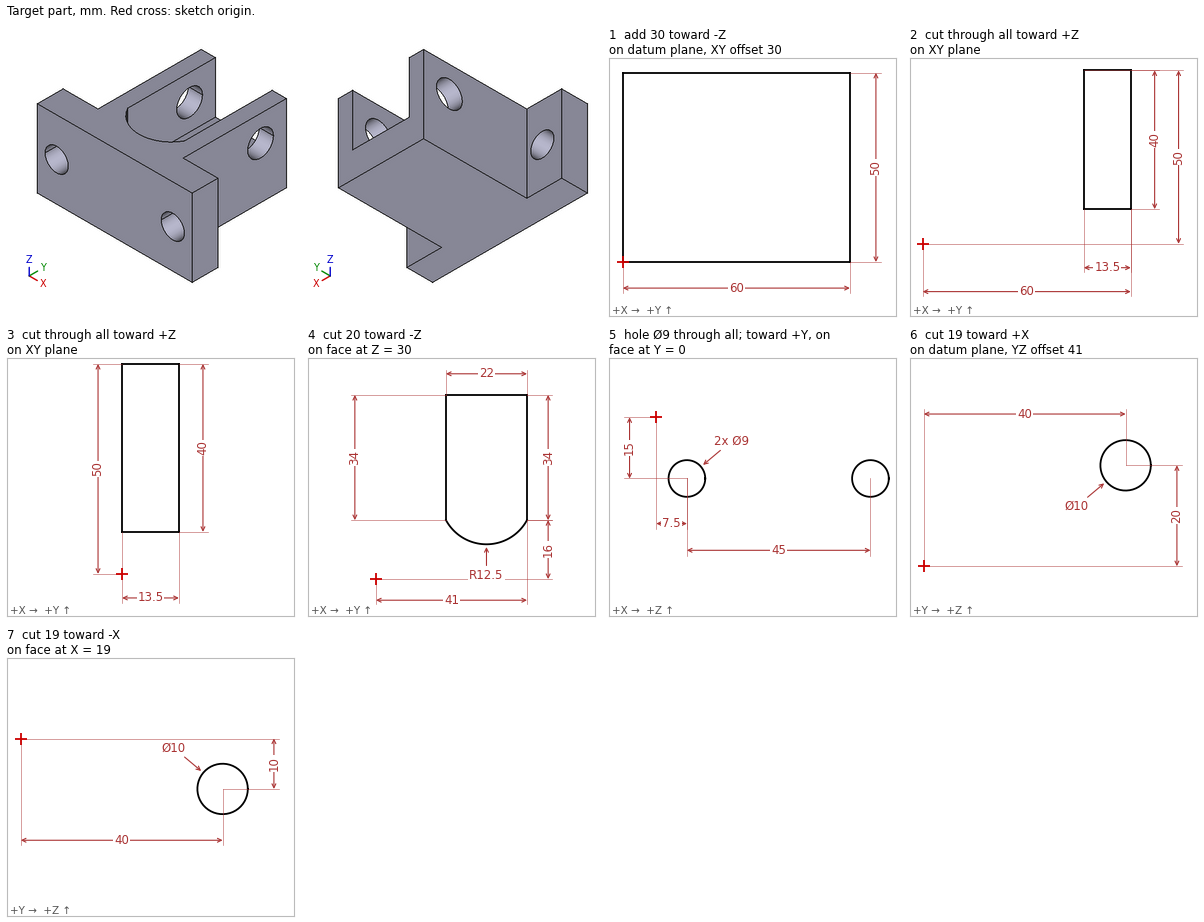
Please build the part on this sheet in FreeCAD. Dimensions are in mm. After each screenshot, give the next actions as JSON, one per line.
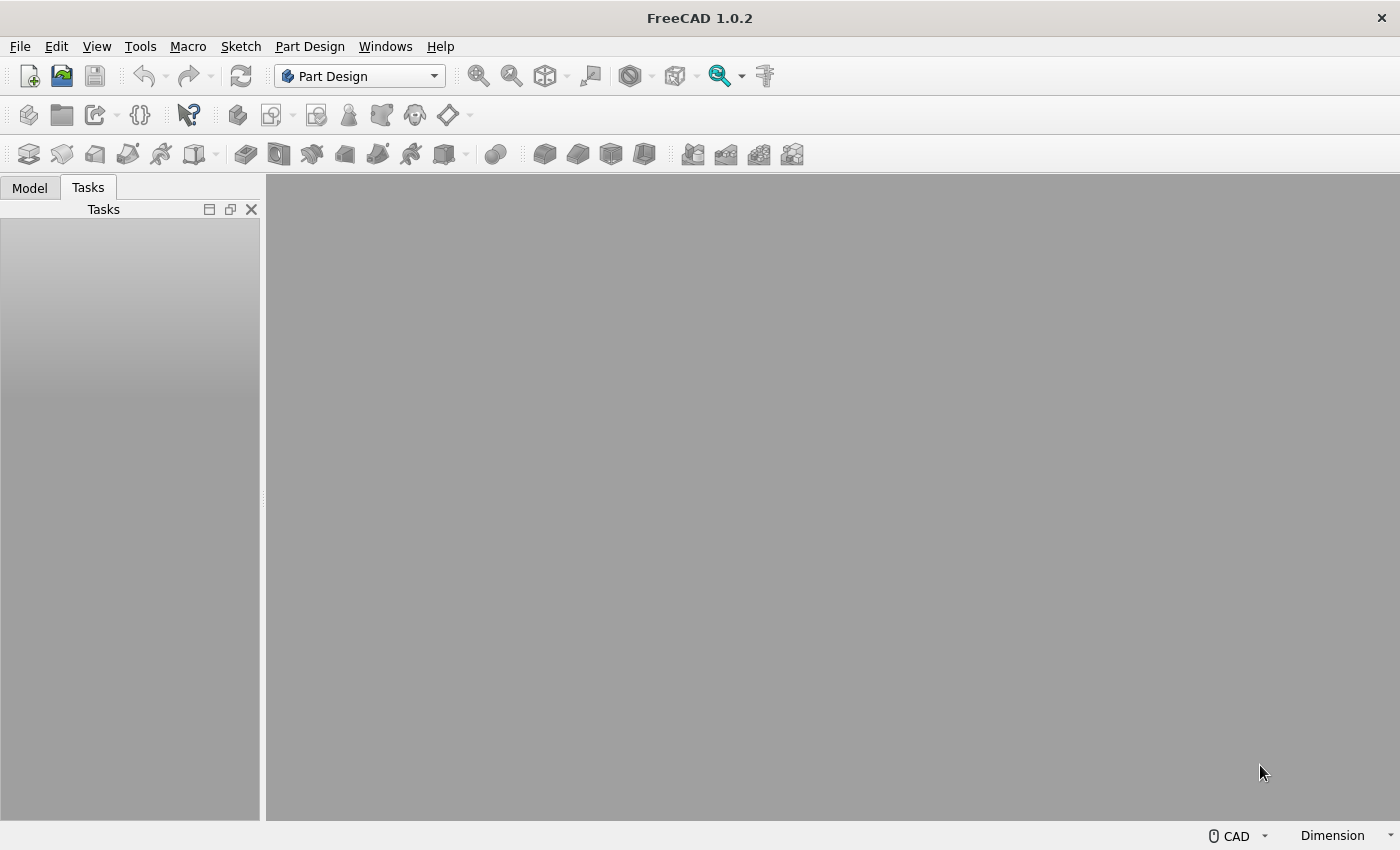
{"action": "key", "text": "ctrl+n"}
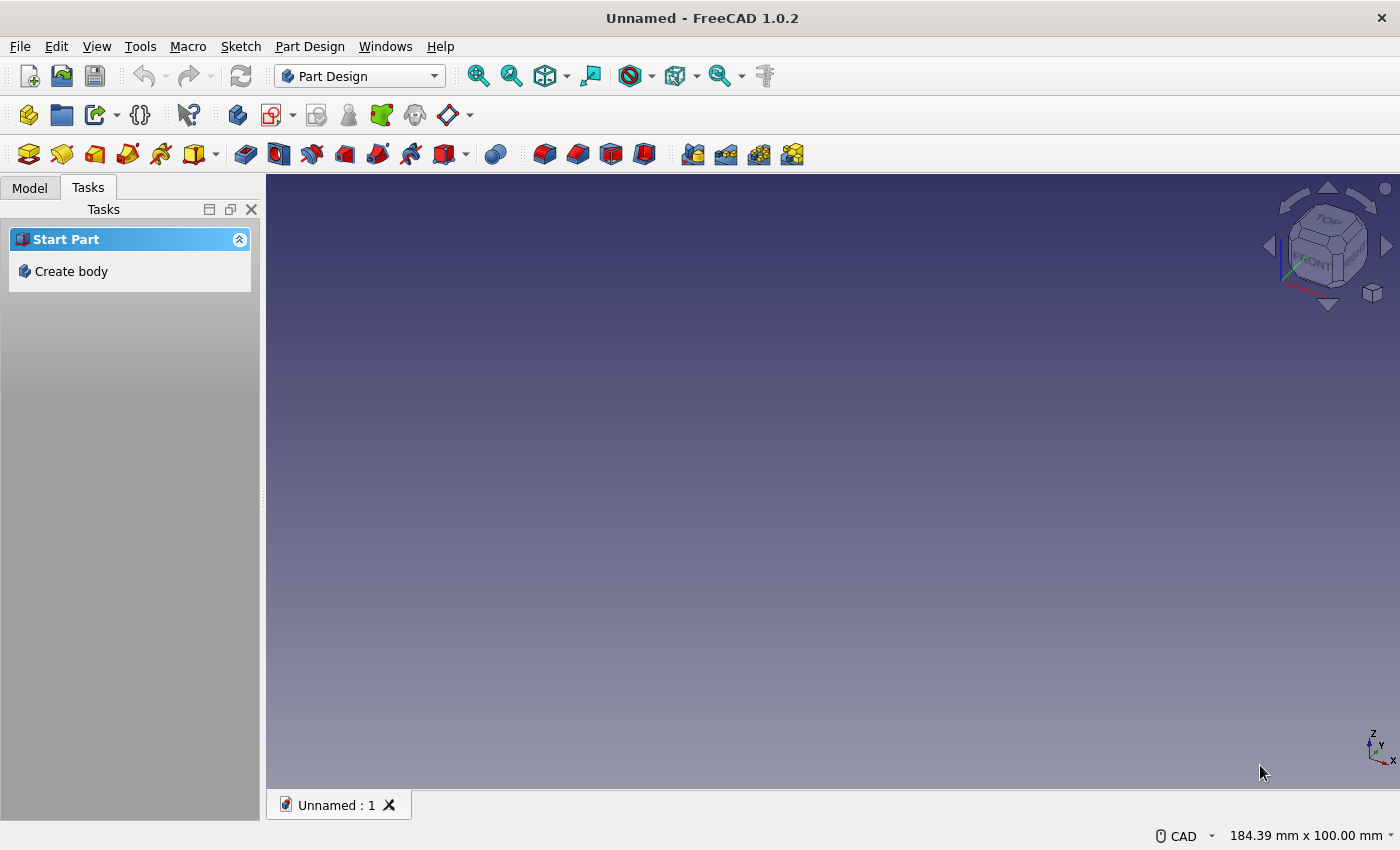
{"action": "left_click", "coordinate": [238, 116]}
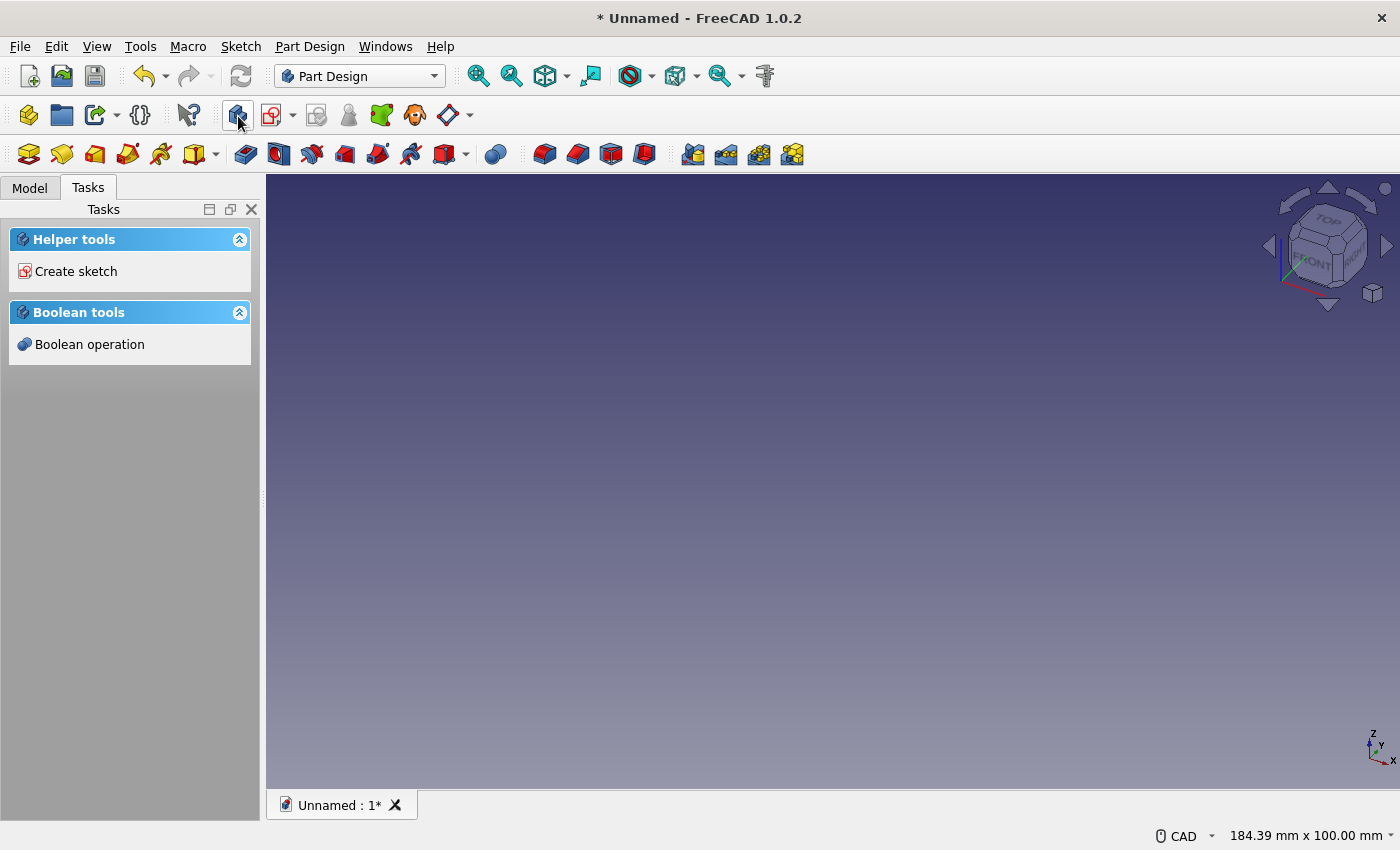
{"action": "left_click", "coordinate": [30, 188]}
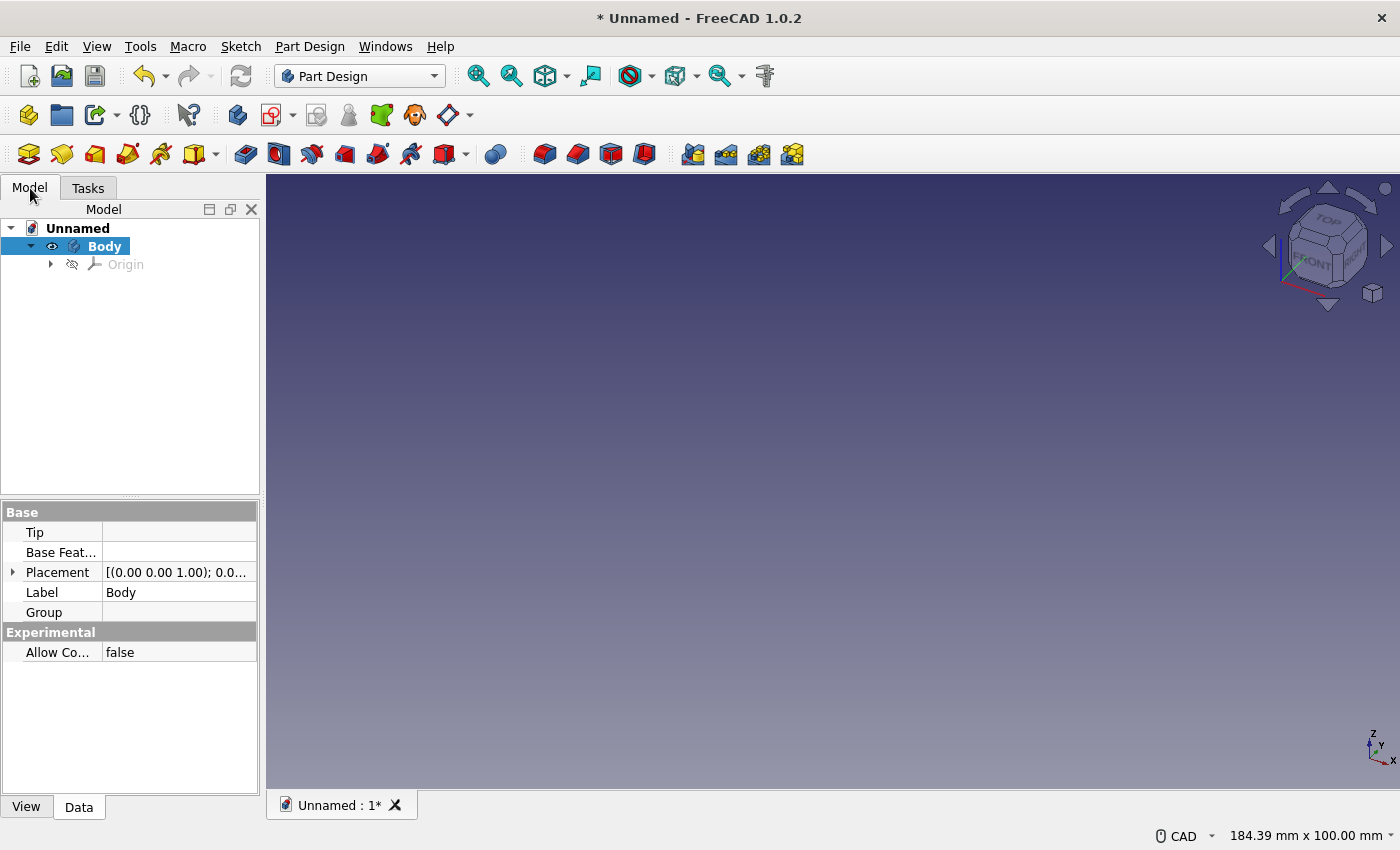
{"action": "left_click", "coordinate": [51, 264]}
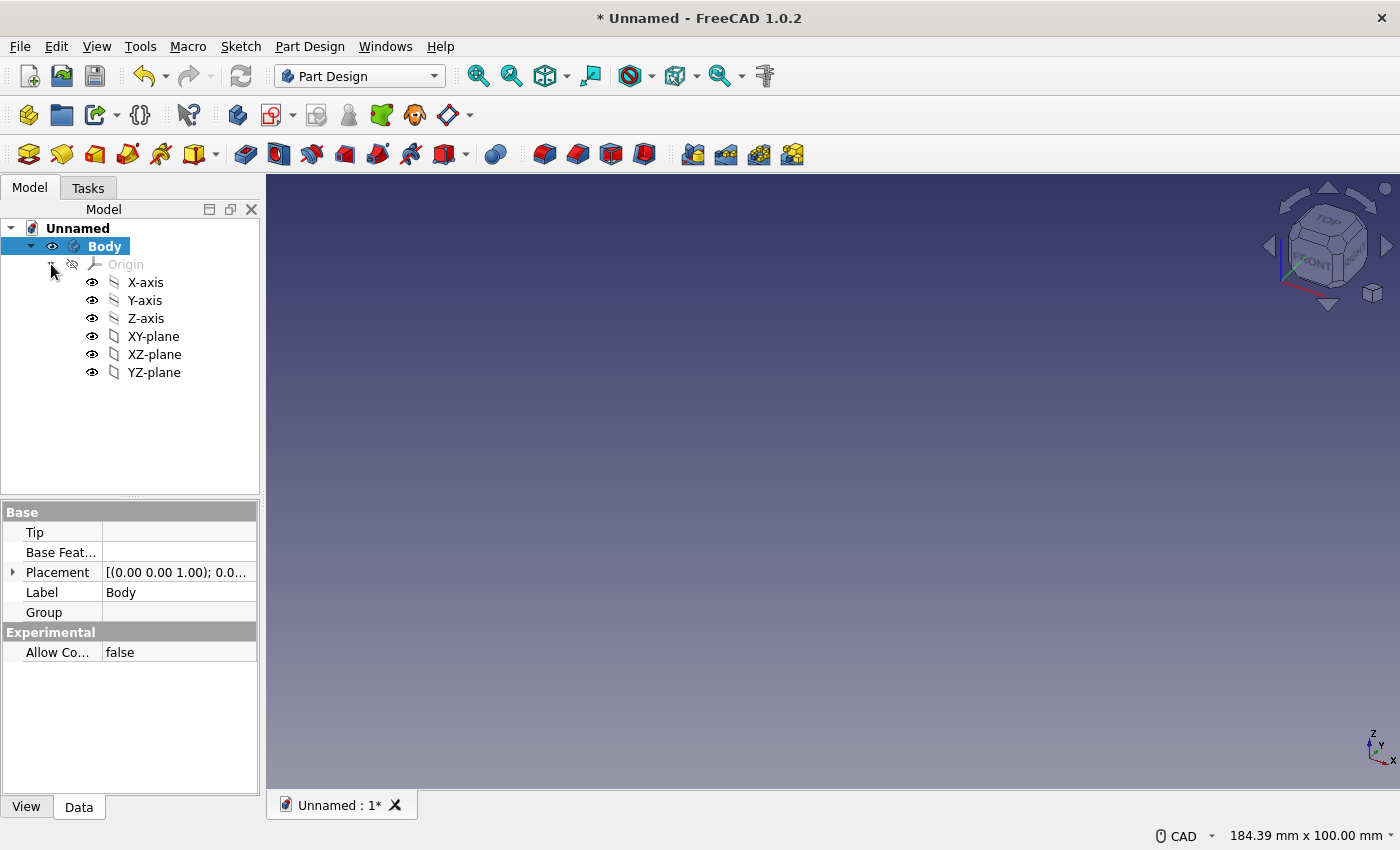
{"action": "left_click", "coordinate": [137, 336]}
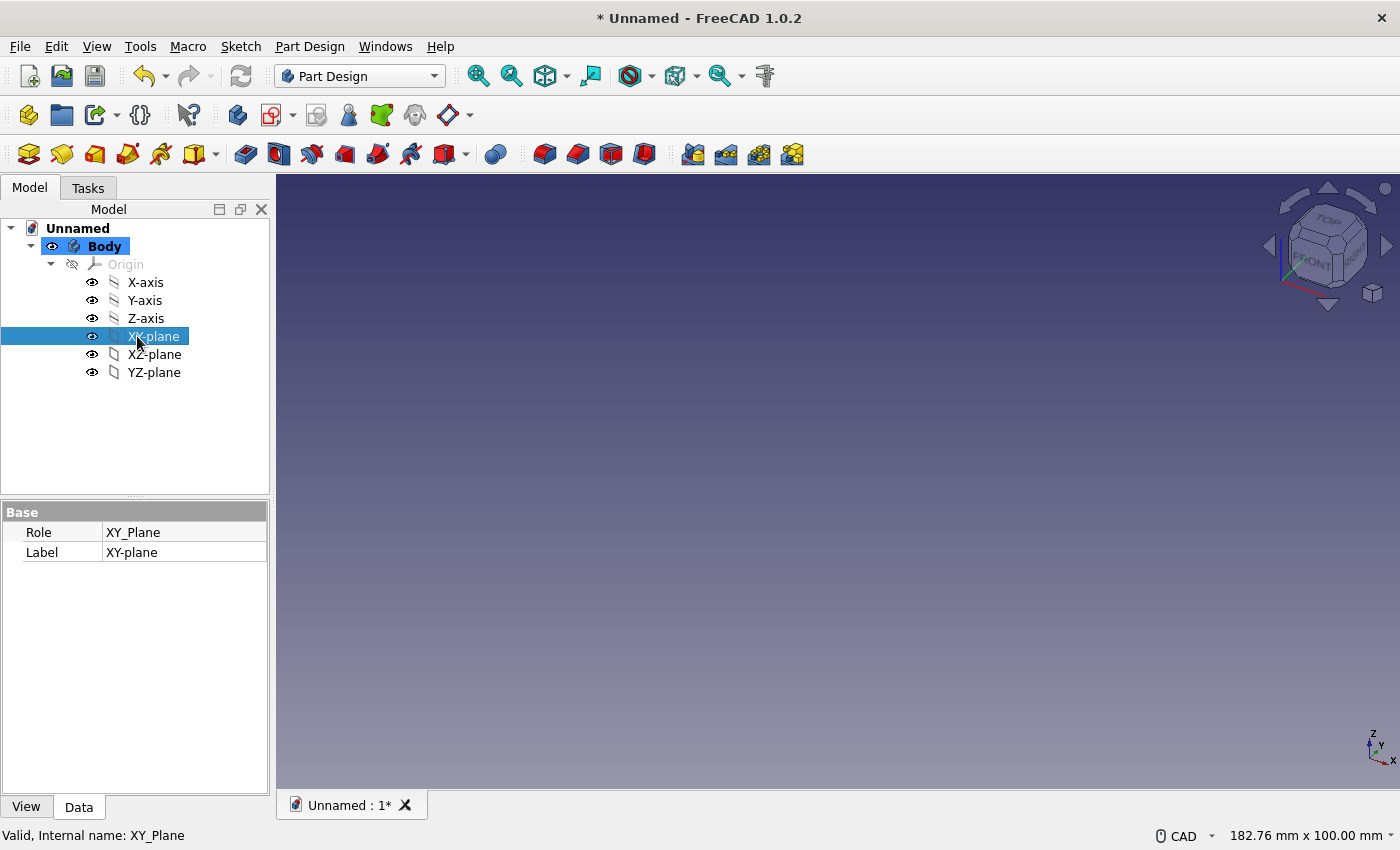
{"action": "left_click", "coordinate": [448, 116]}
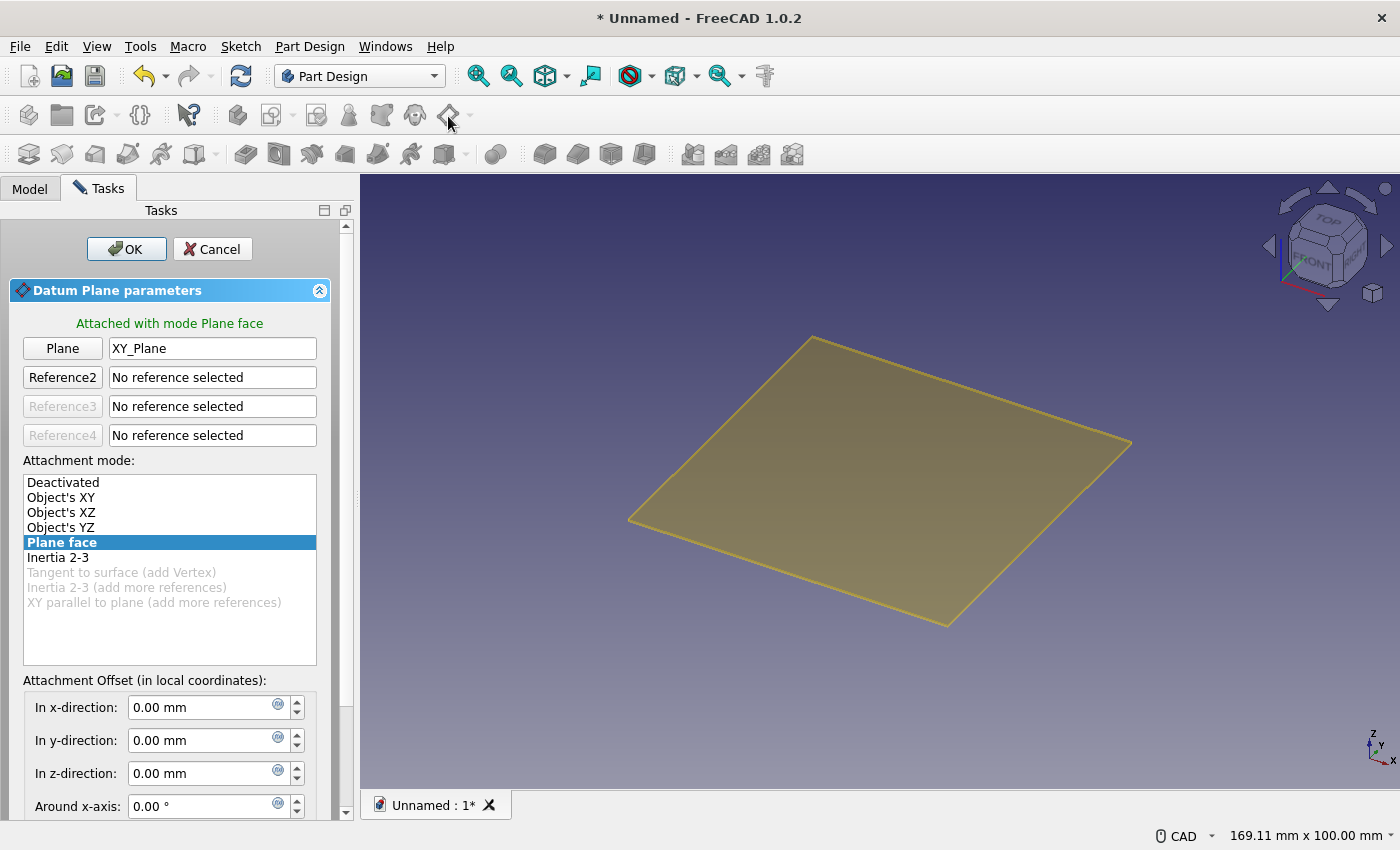
{"action": "triple_click", "coordinate": [210, 774]}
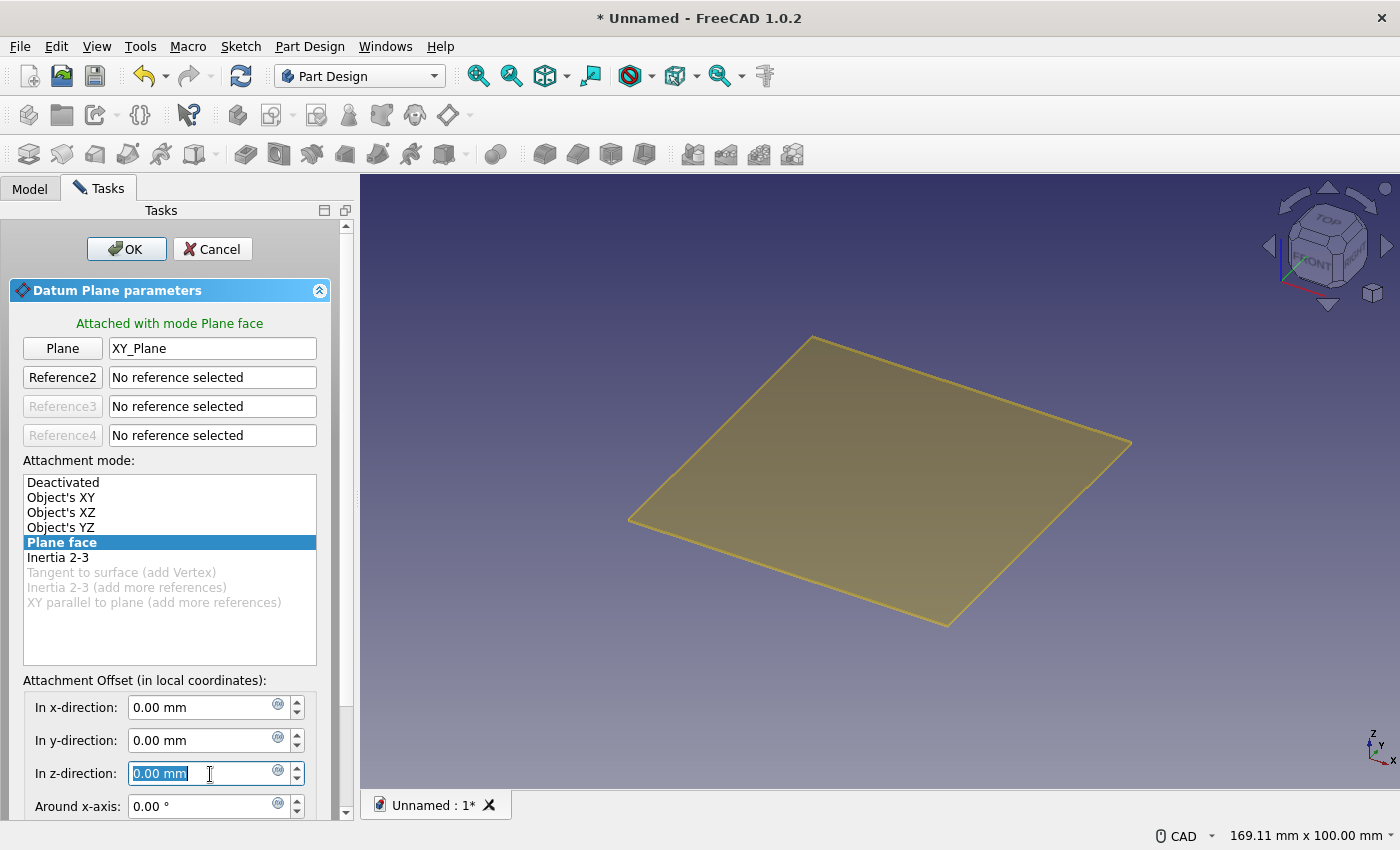
{"action": "type", "text": "30"}
{"action": "key", "text": "Tab"}